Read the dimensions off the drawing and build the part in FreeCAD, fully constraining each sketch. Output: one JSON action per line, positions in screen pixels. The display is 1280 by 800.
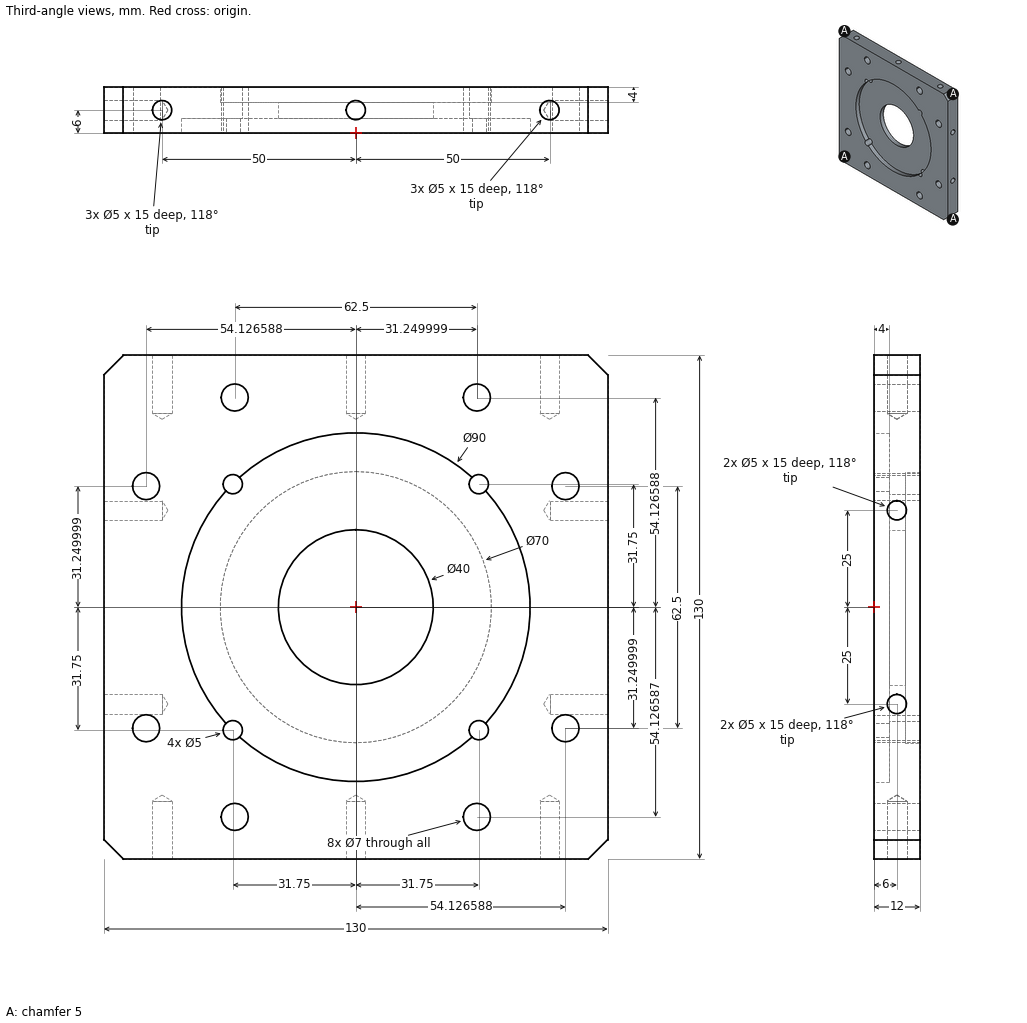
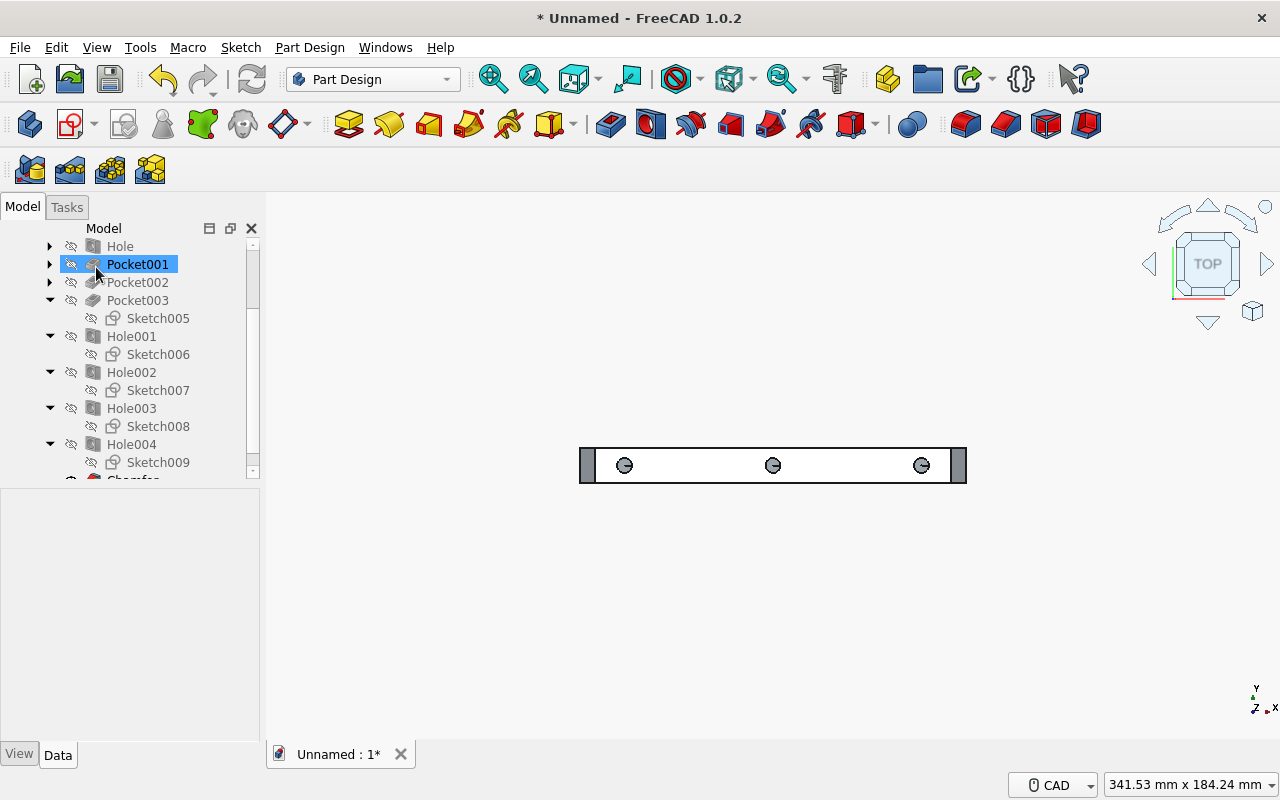
{"action": "key", "text": "0"}